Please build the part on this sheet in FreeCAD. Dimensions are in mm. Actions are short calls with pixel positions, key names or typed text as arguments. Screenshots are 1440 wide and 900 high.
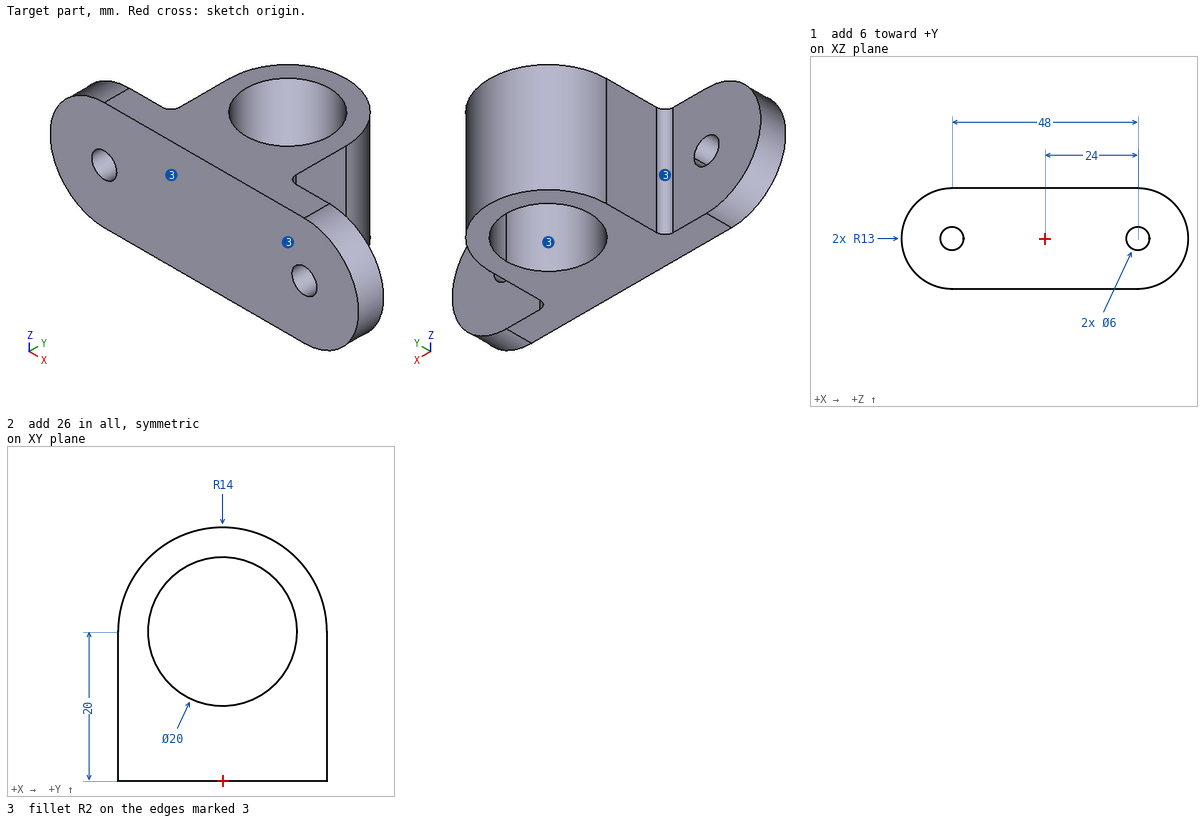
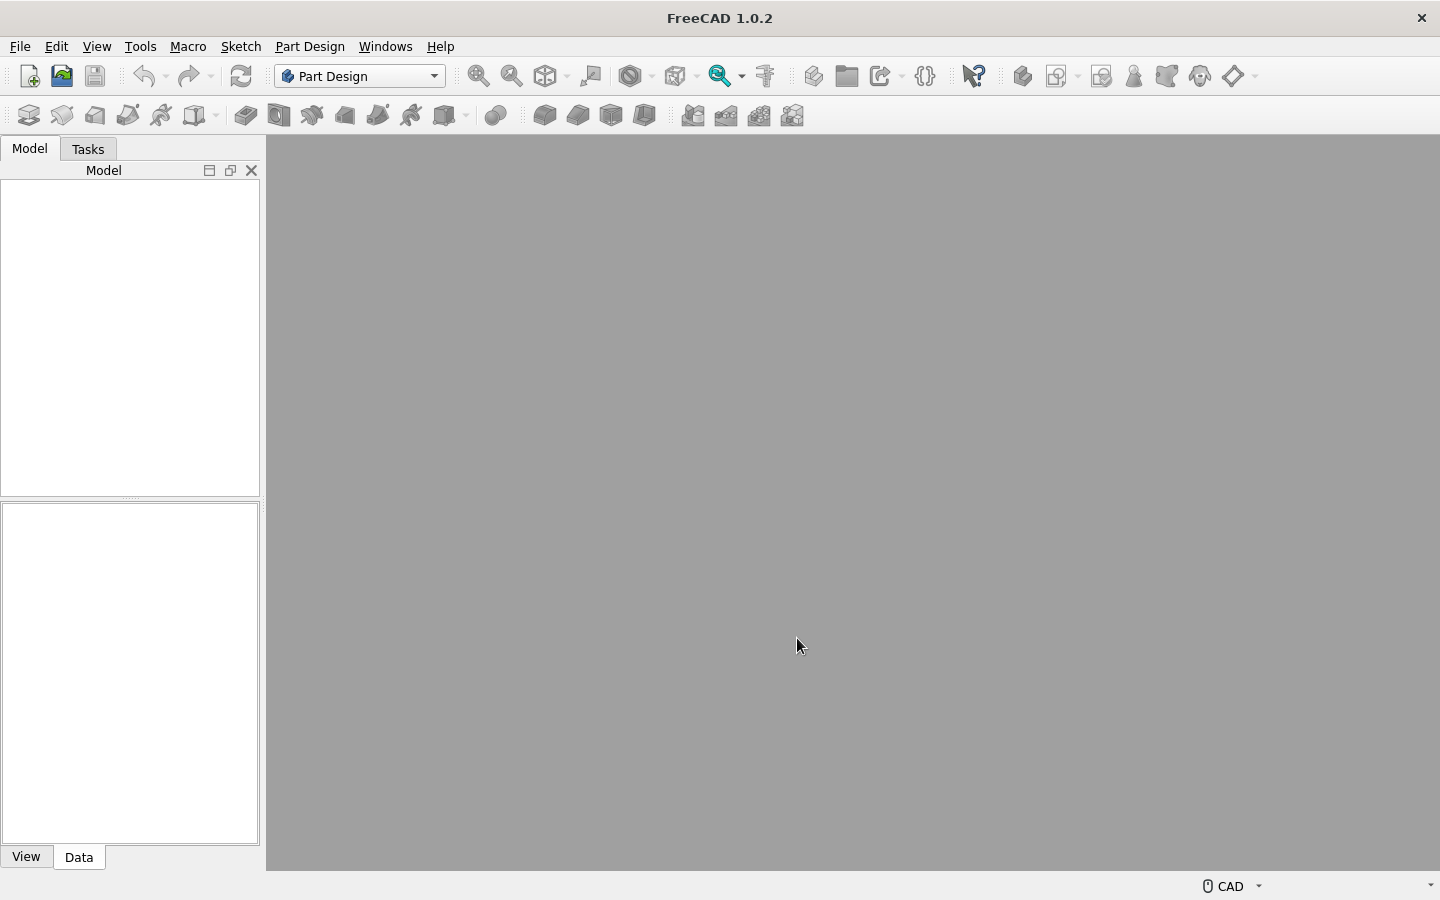
key(ctrl+n)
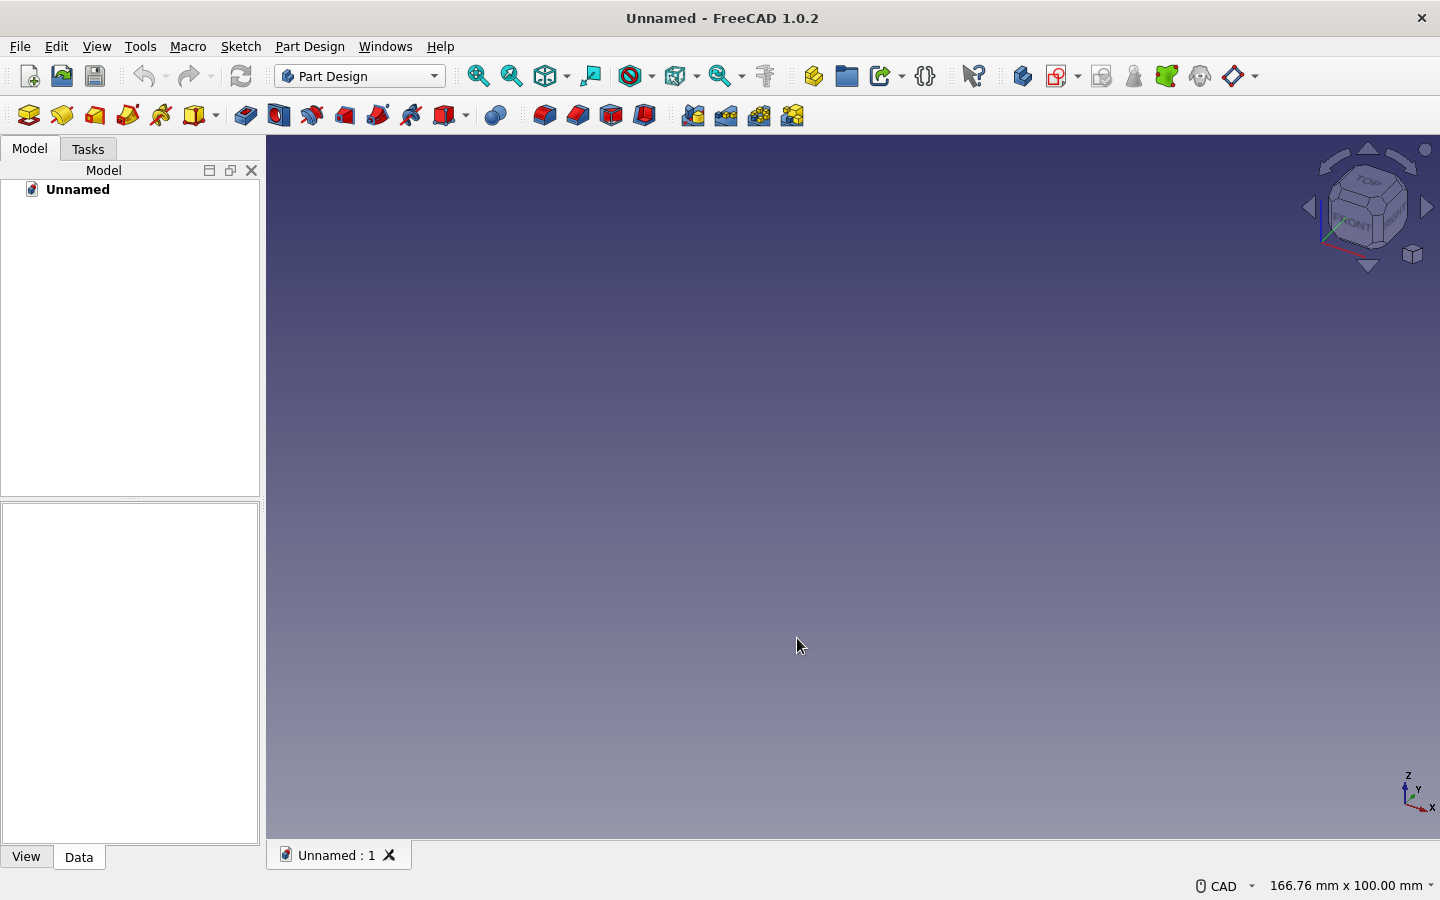
click(1056, 76)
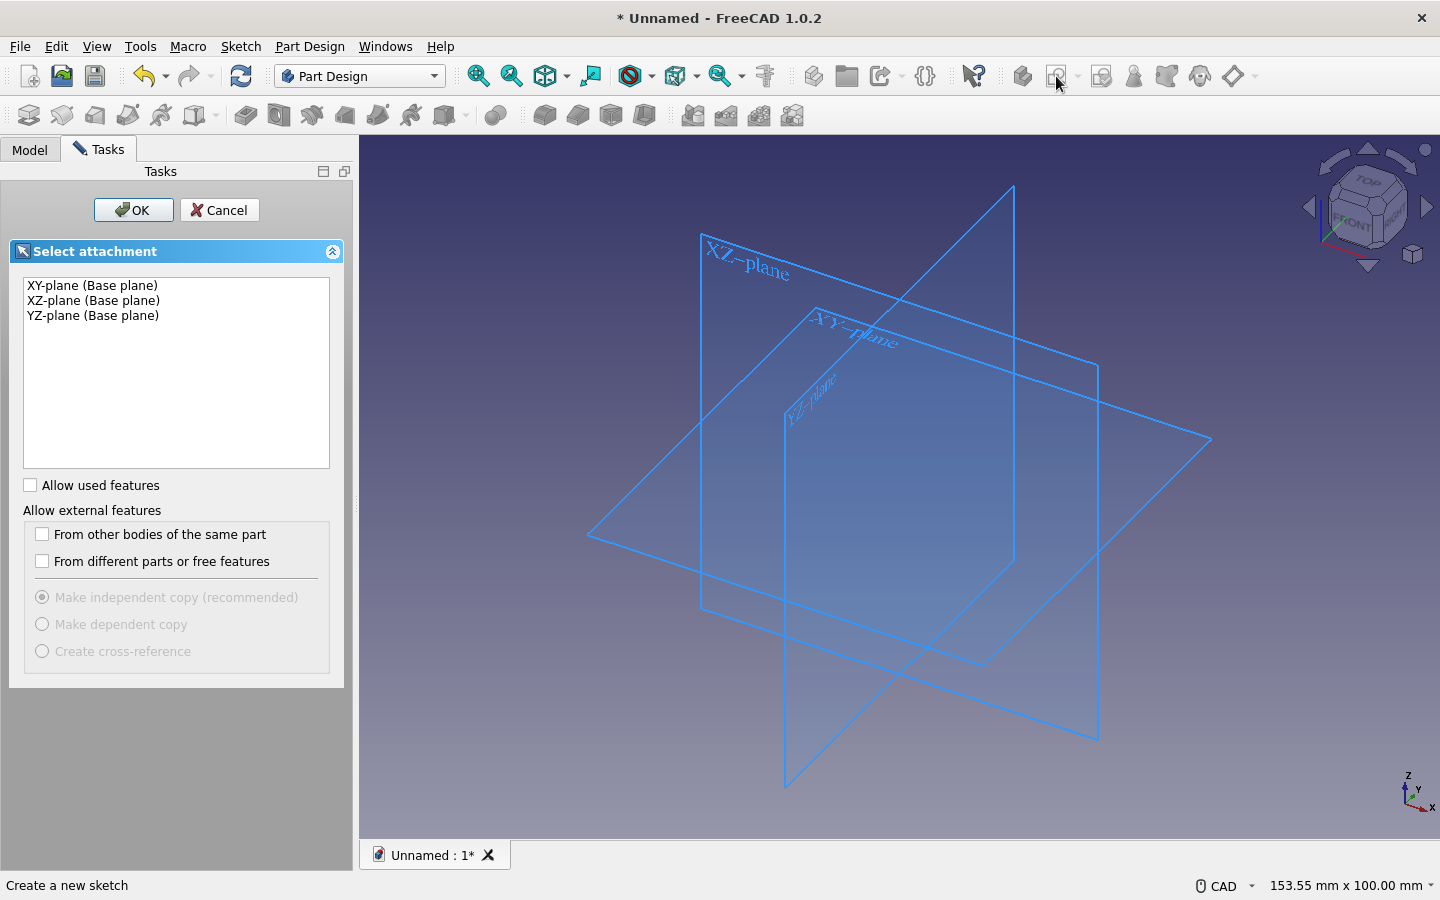
click(84, 300)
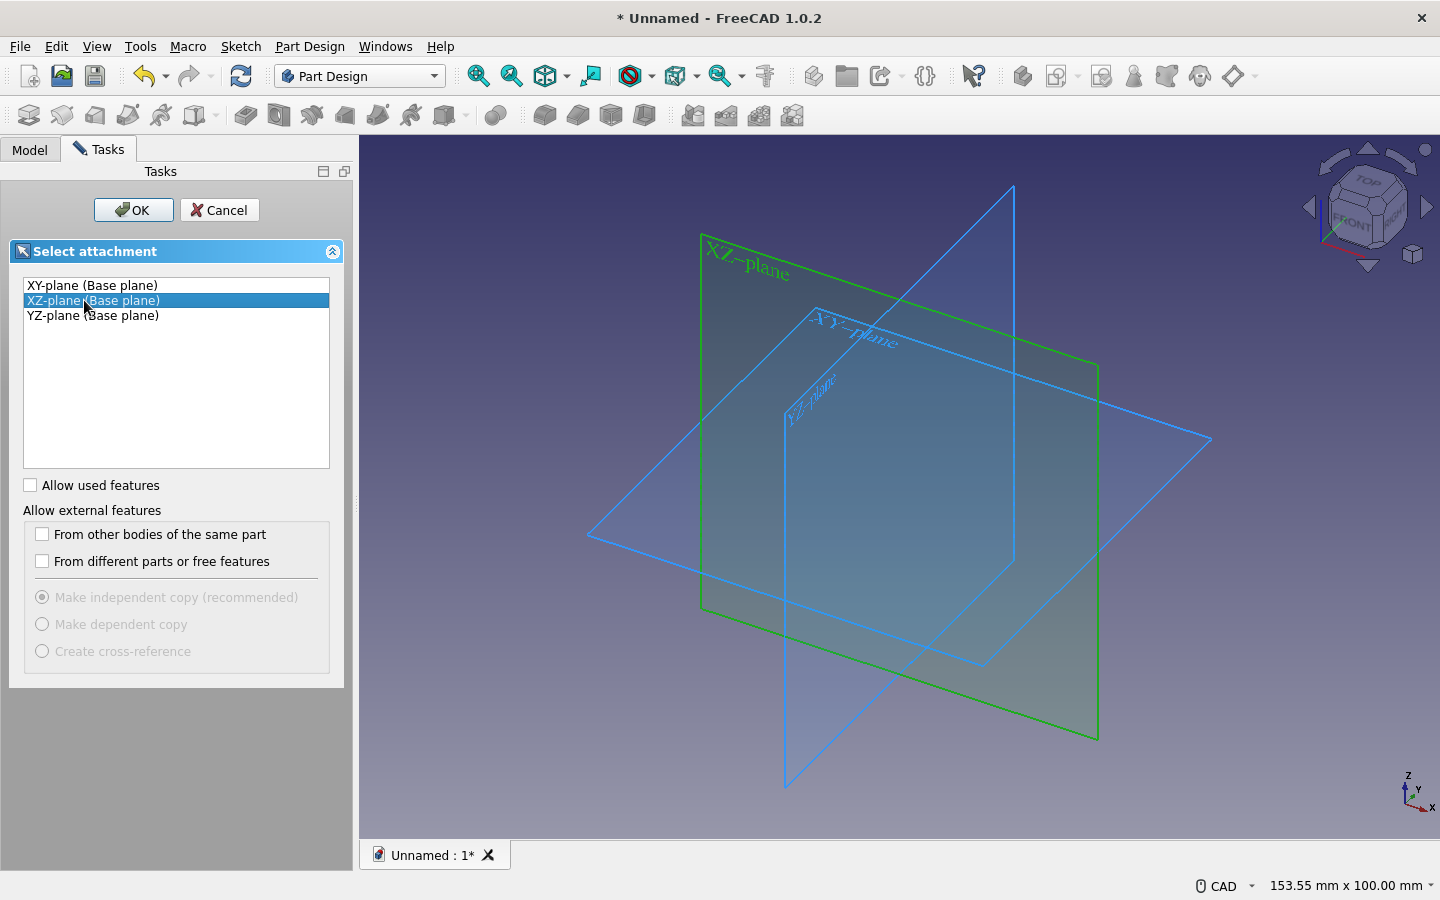
click(134, 210)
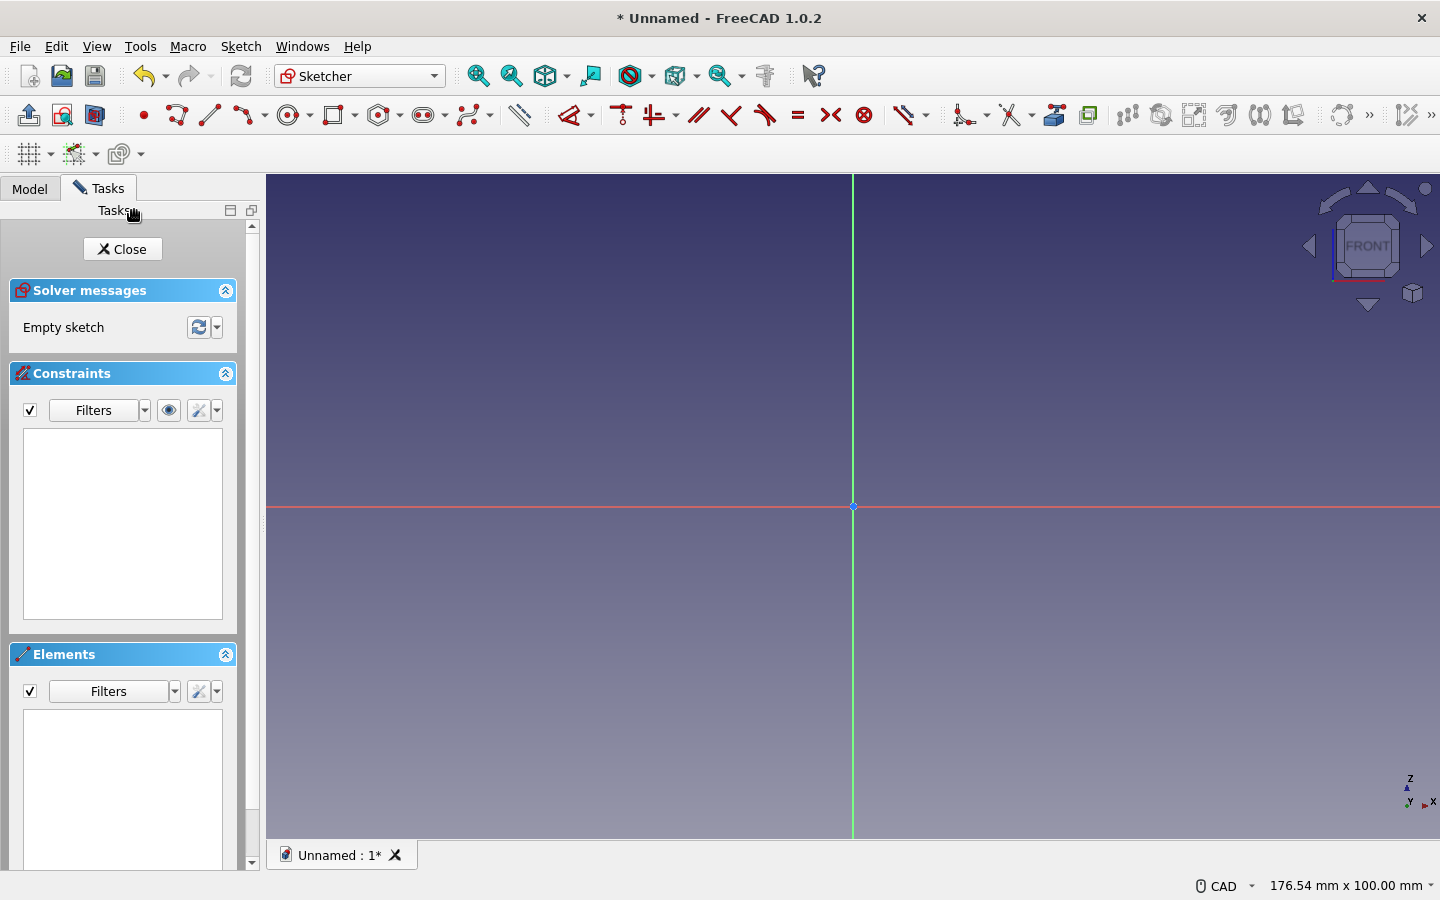
scroll(992, 506, up, 2)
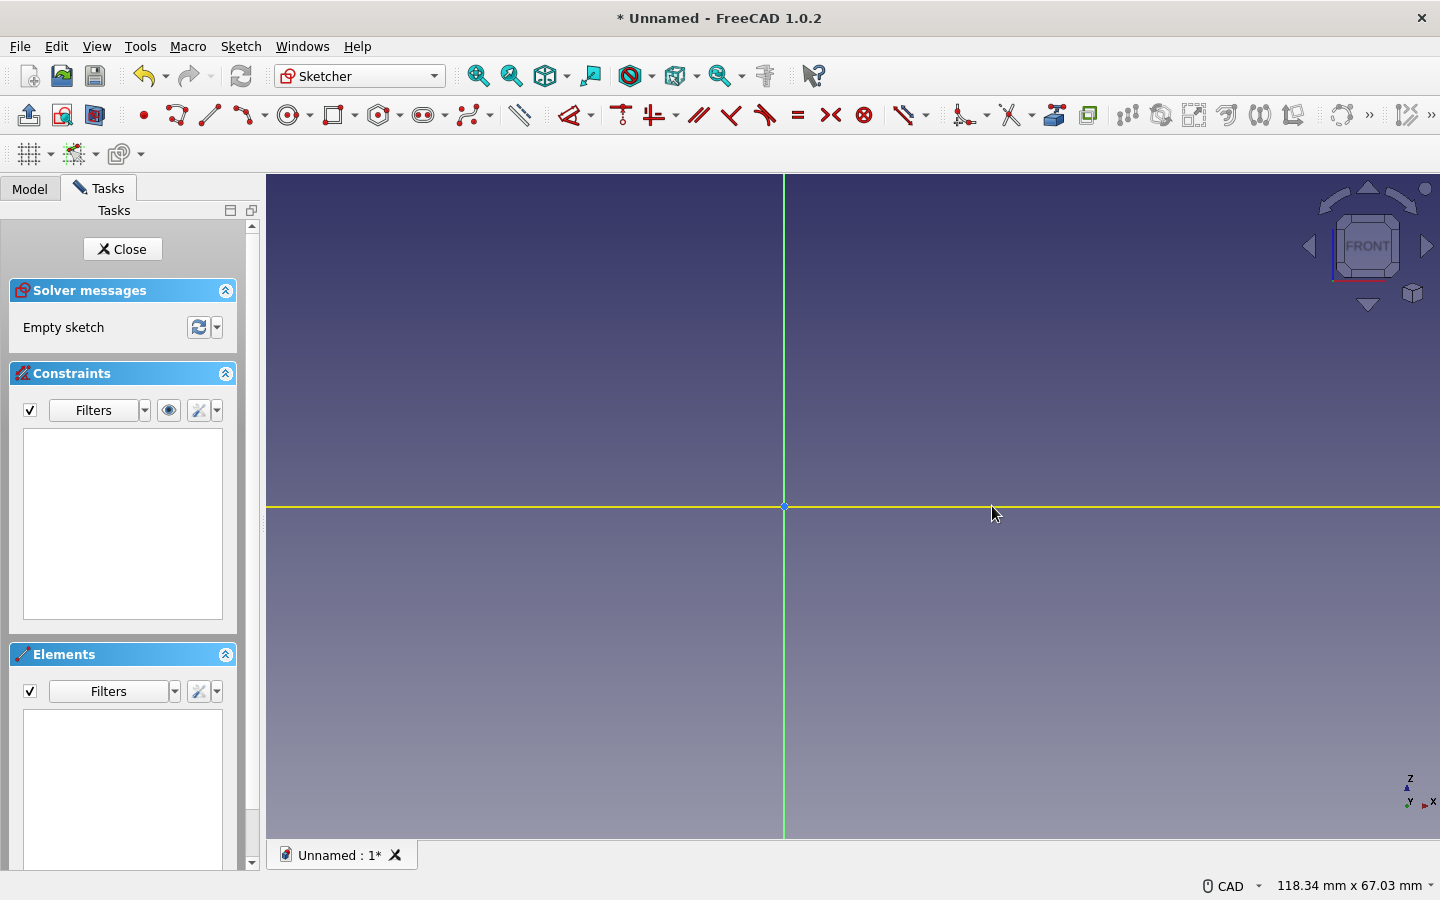
key(g)
key(s)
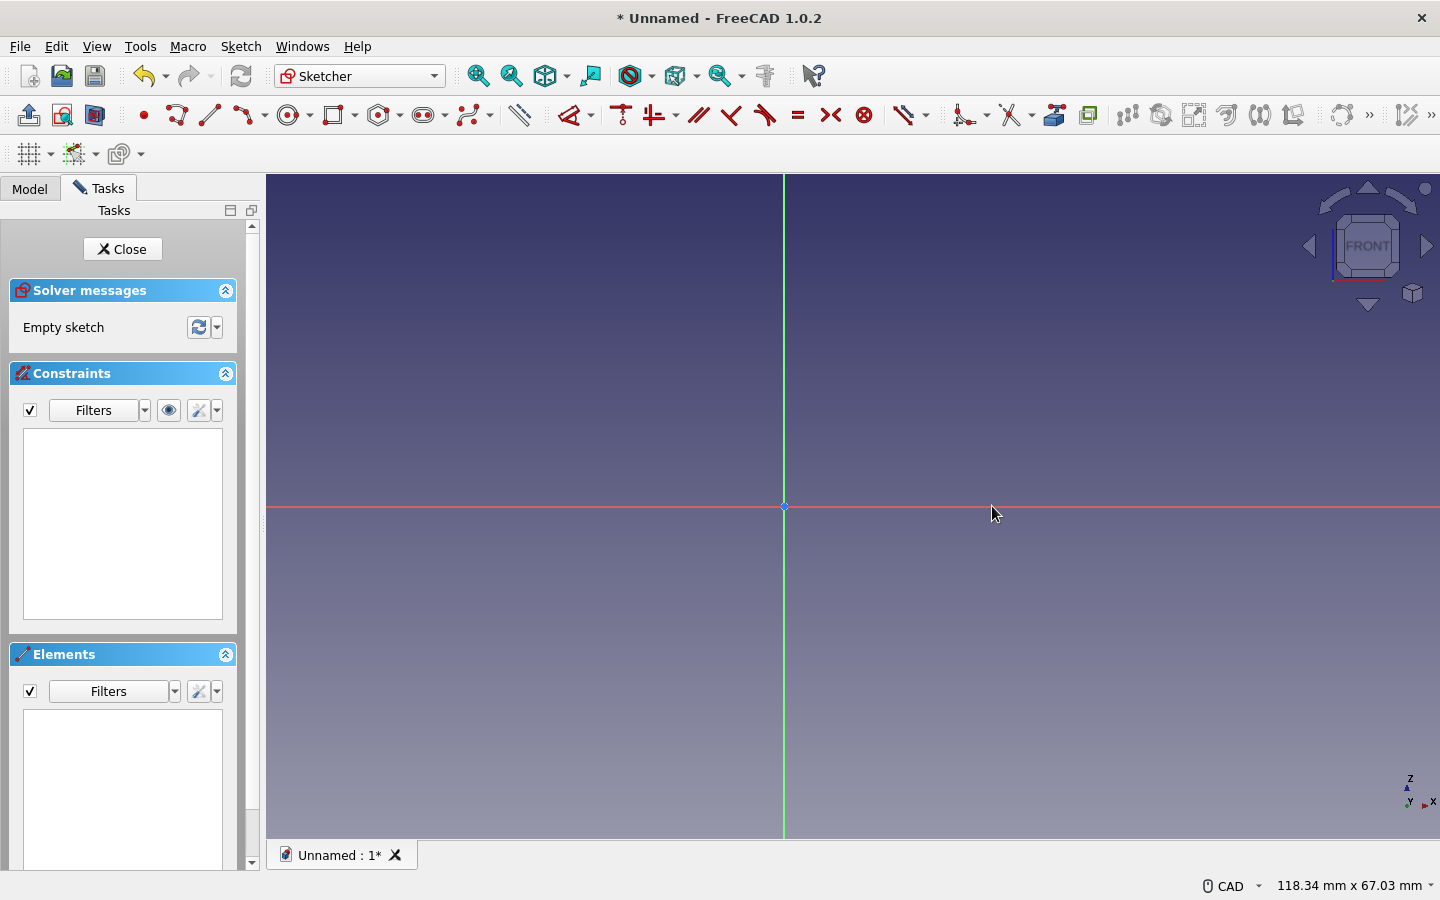
click(546, 506)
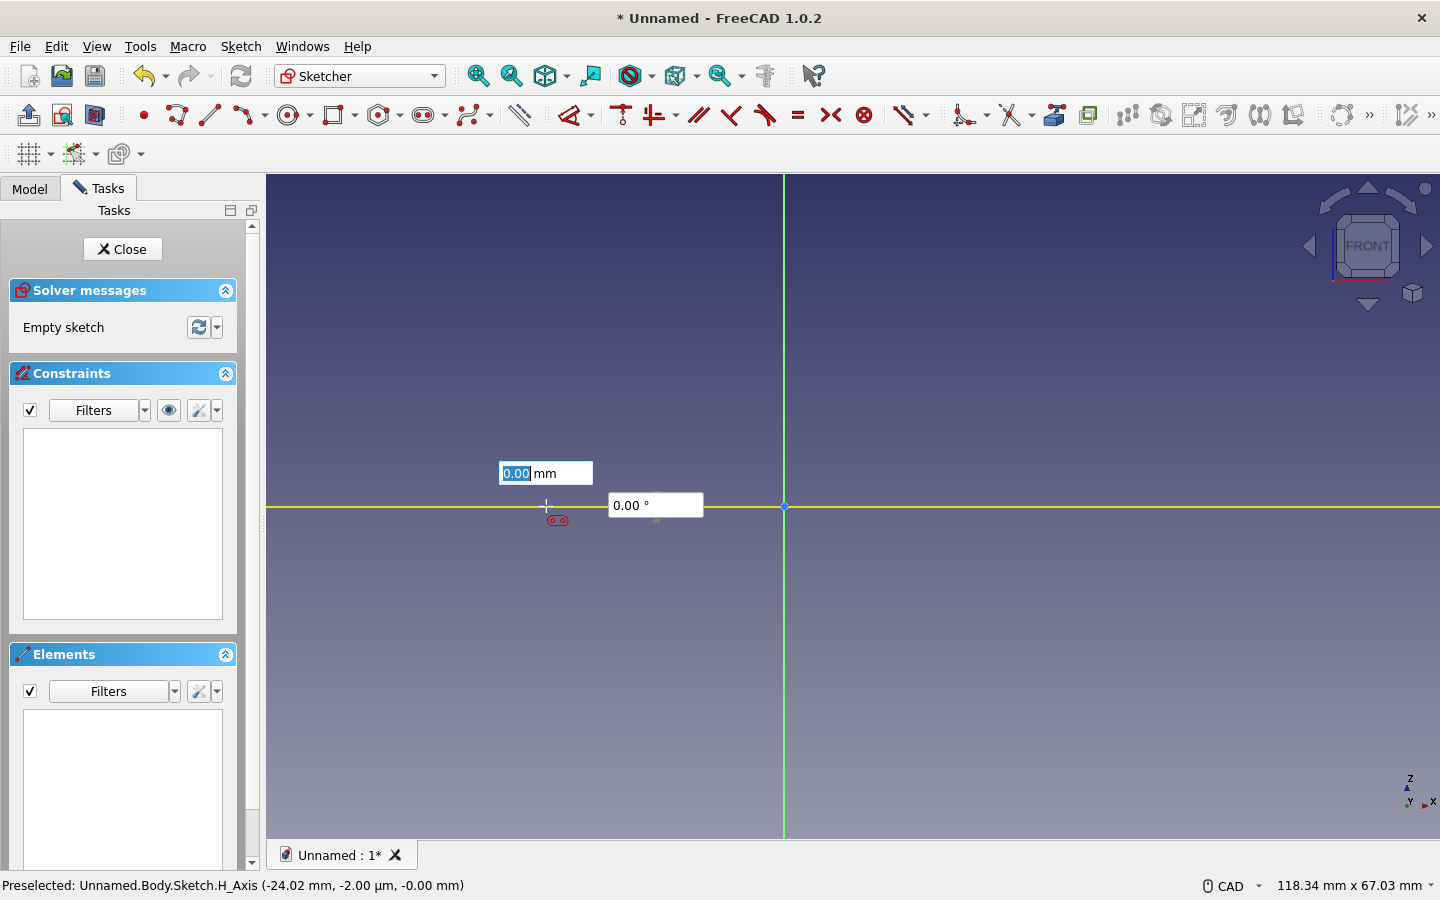
click(1022, 498)